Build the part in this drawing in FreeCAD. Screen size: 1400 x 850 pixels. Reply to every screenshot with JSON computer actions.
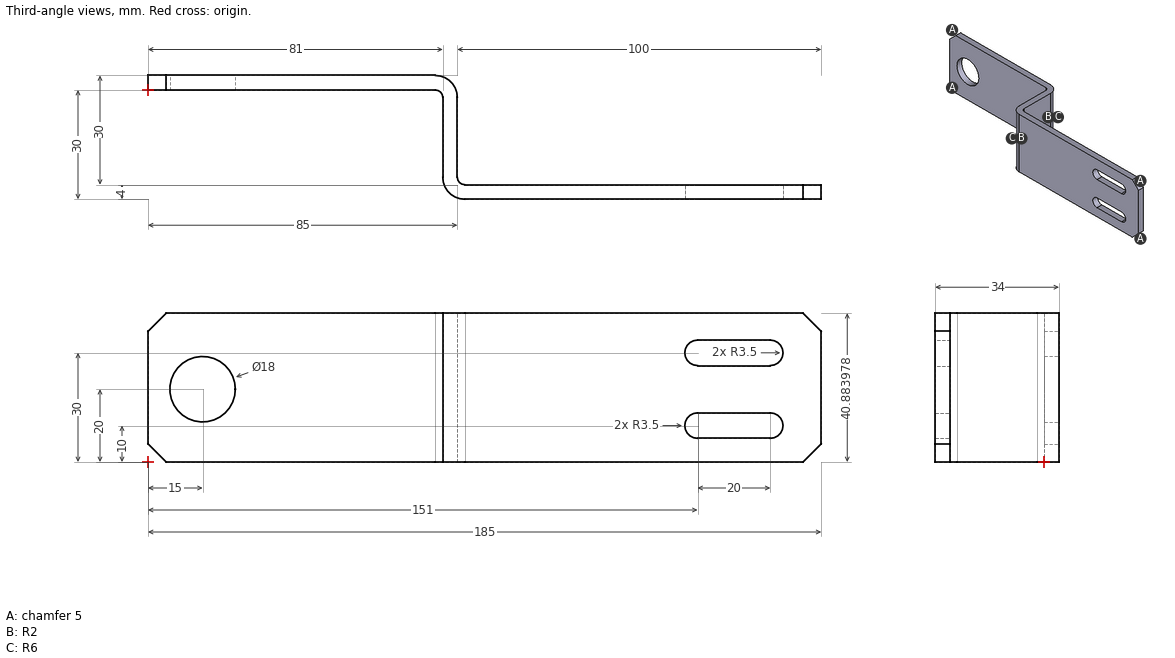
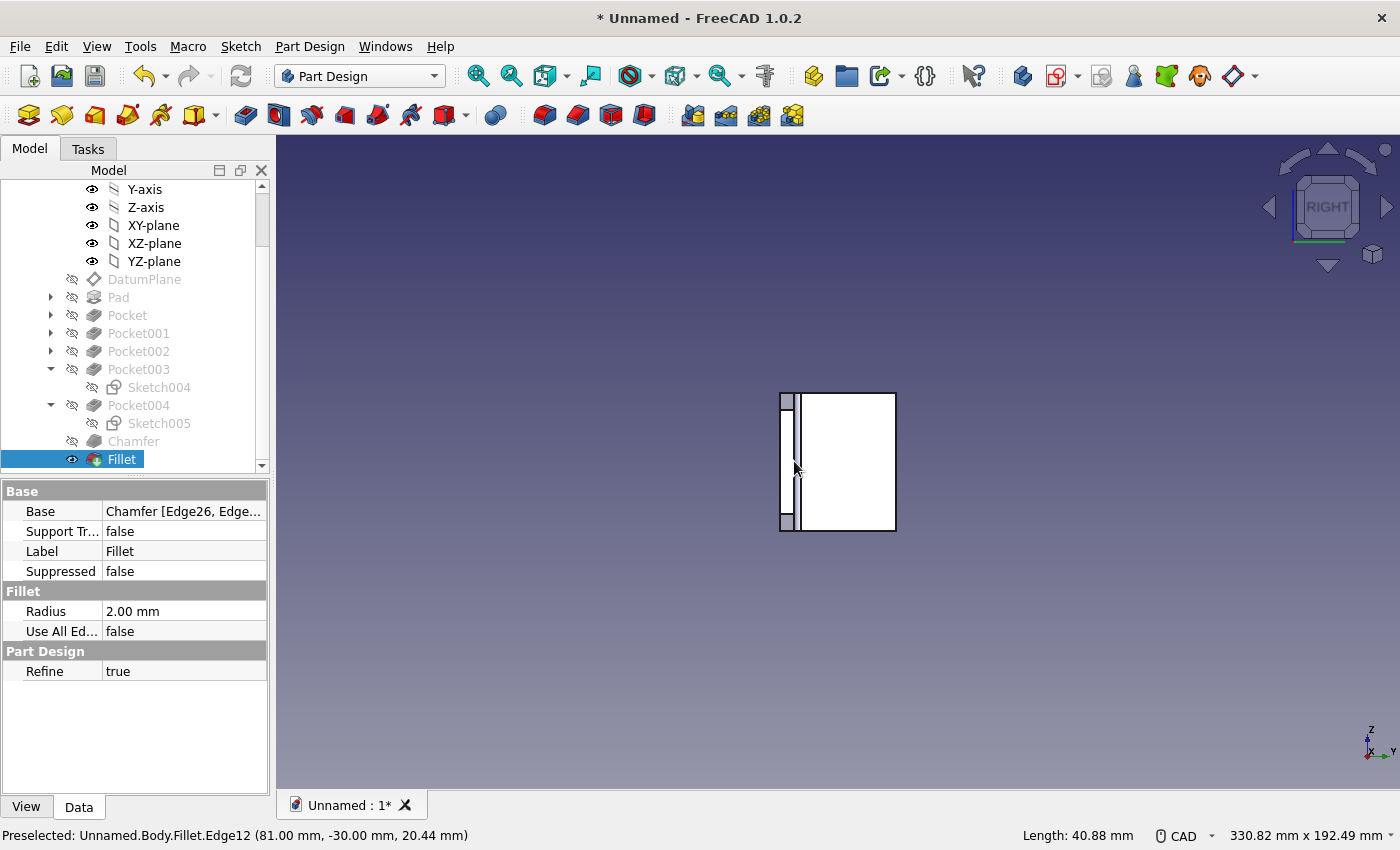
{"action": "left_click", "coordinate": [479, 76]}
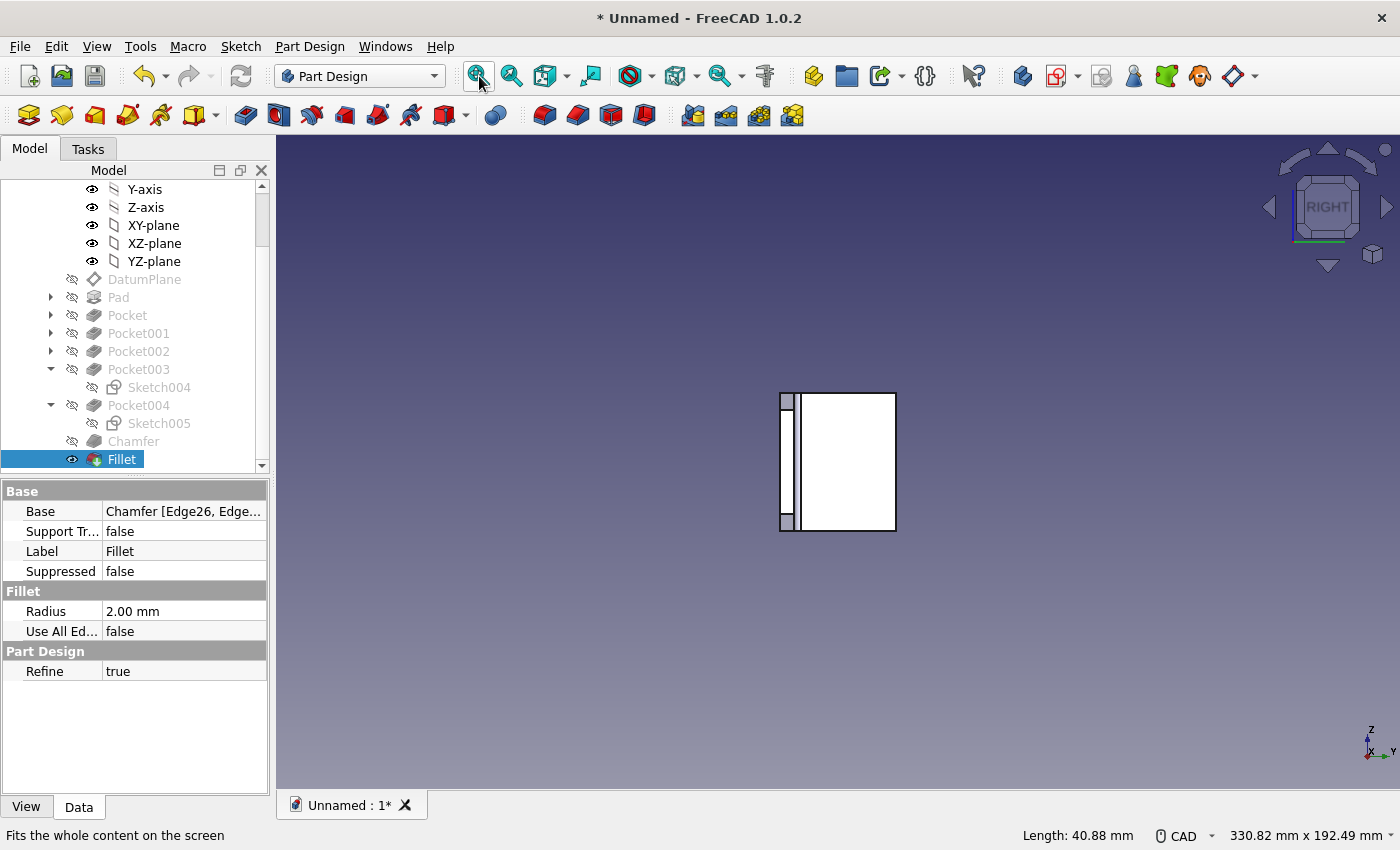
{"action": "left_click", "coordinate": [896, 461], "text": "ctrl"}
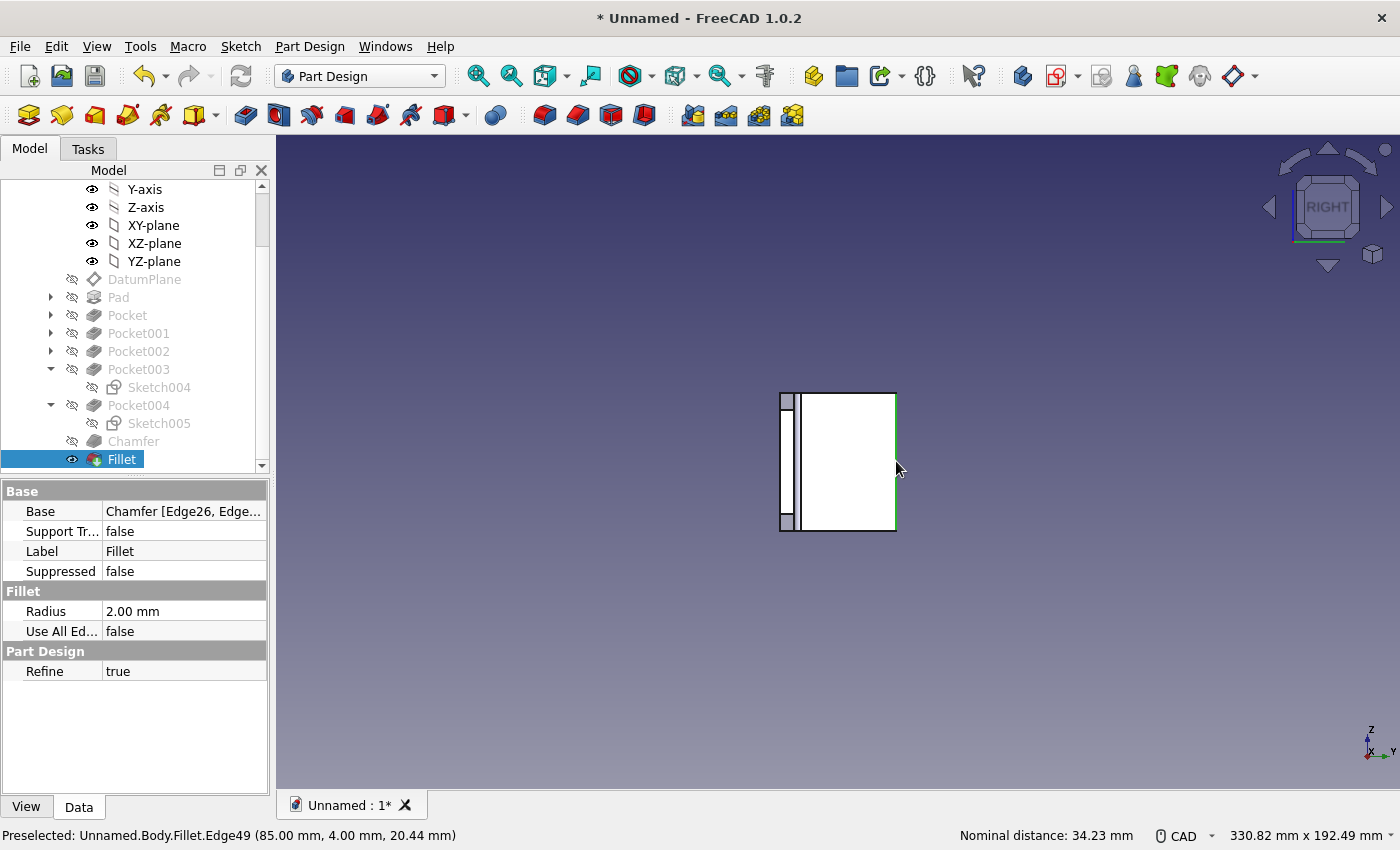
{"action": "left_click", "coordinate": [545, 116]}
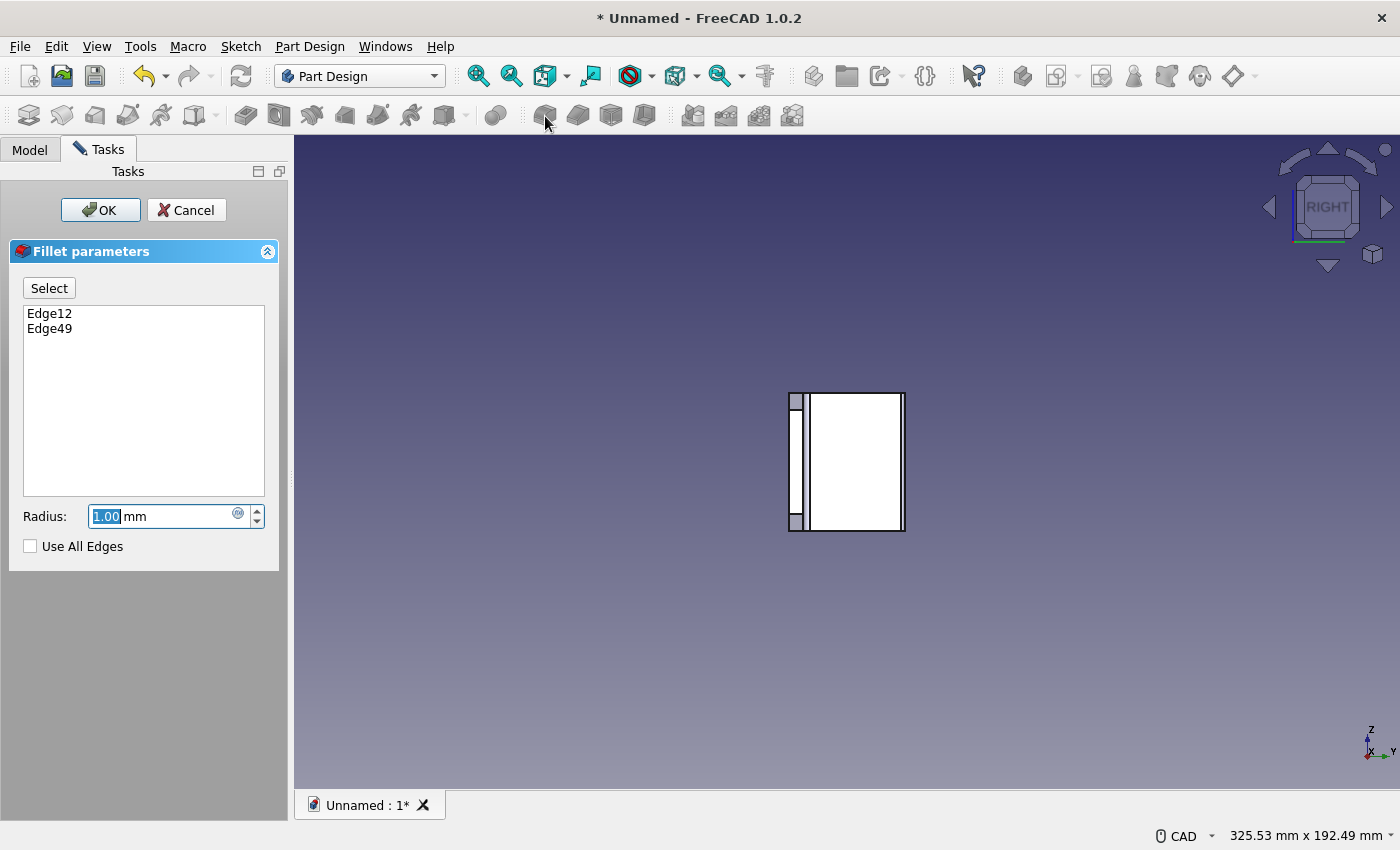
{"action": "type", "text": "6"}
{"action": "key", "text": "Tab"}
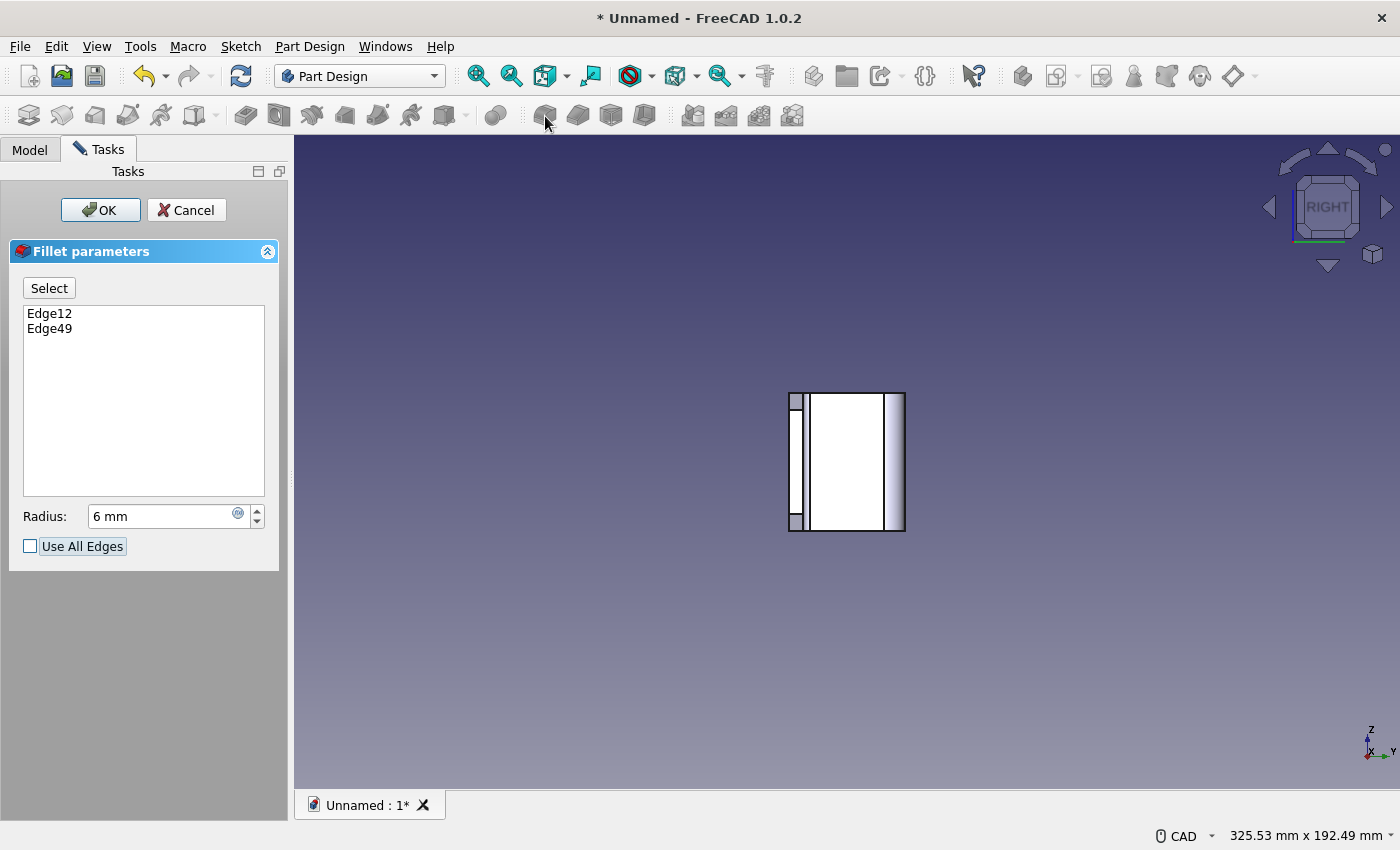
{"action": "left_click", "coordinate": [101, 210]}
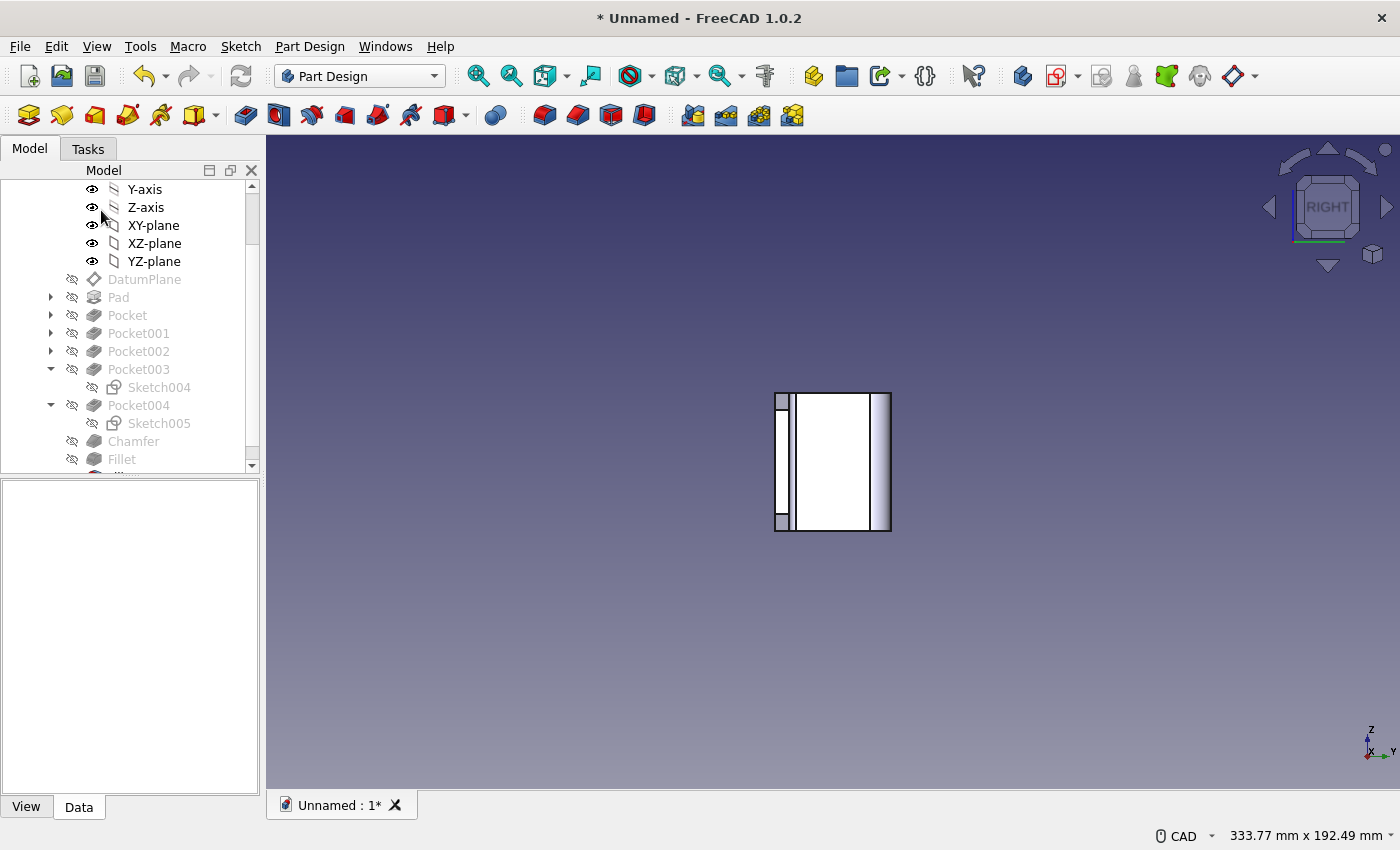
{"action": "key", "text": "0"}